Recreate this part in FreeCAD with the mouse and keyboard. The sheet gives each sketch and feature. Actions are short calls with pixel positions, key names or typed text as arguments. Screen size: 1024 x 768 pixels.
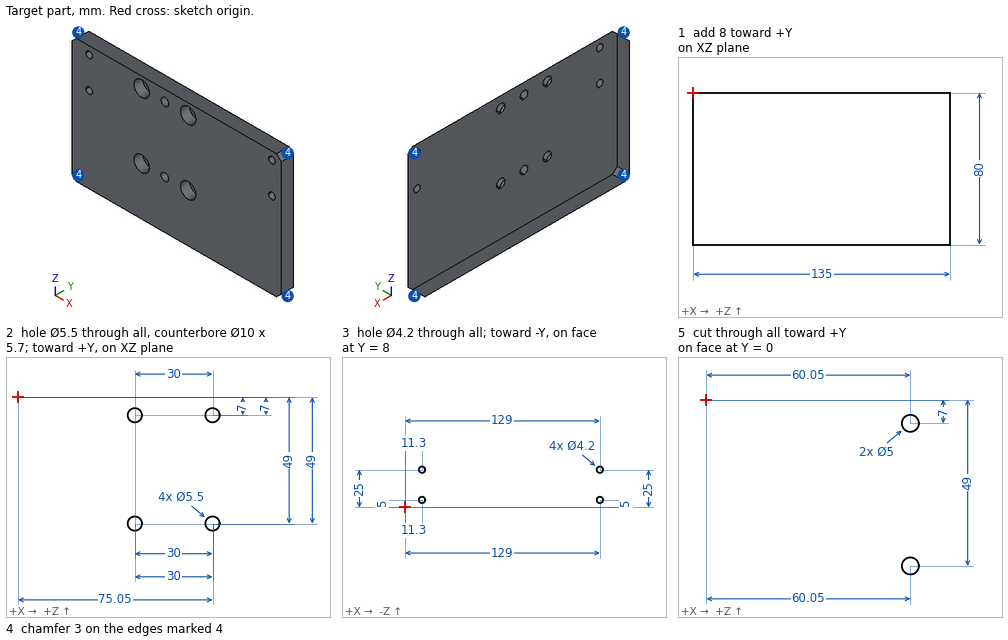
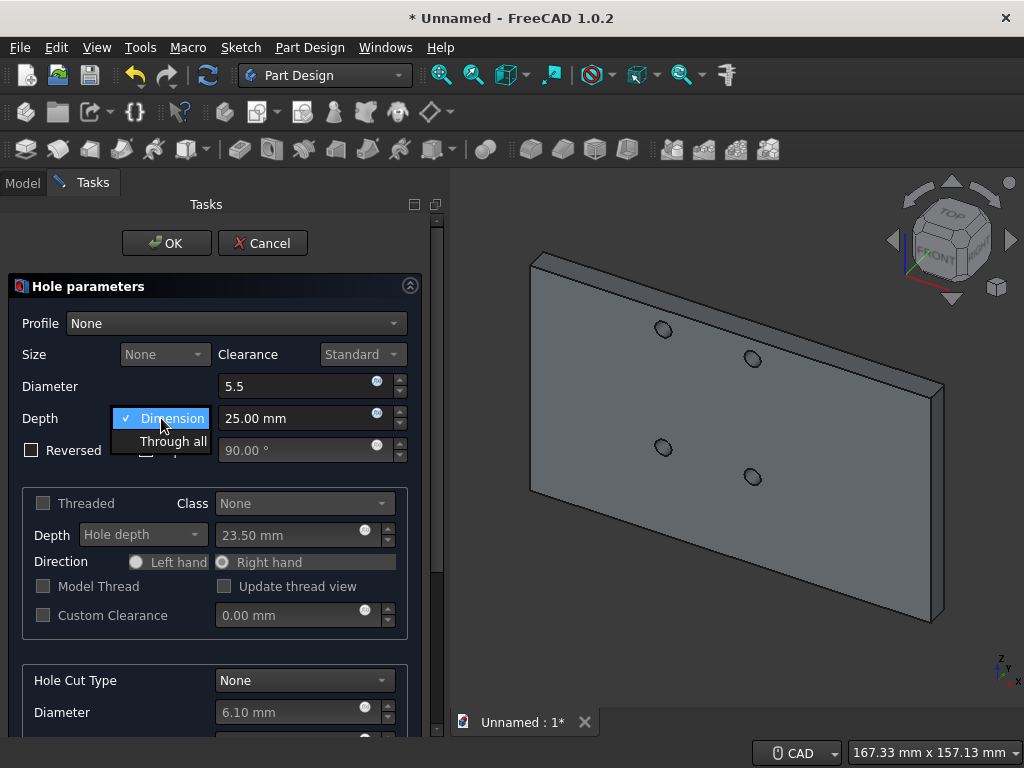
click(160, 442)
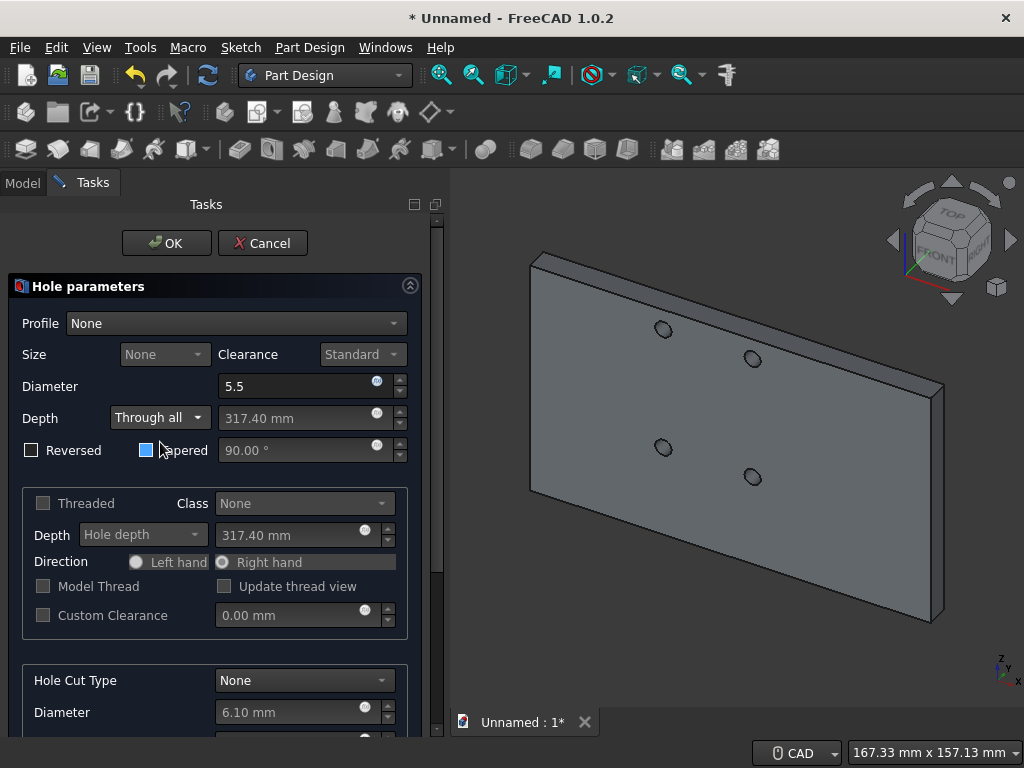
click(306, 680)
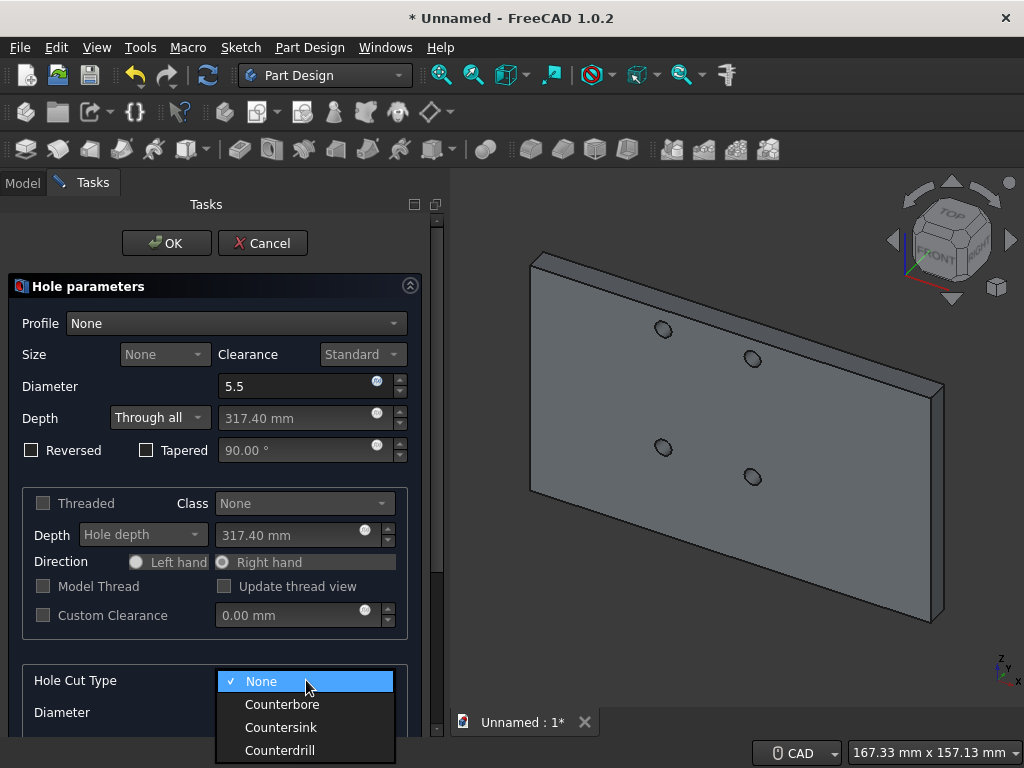
click(304, 704)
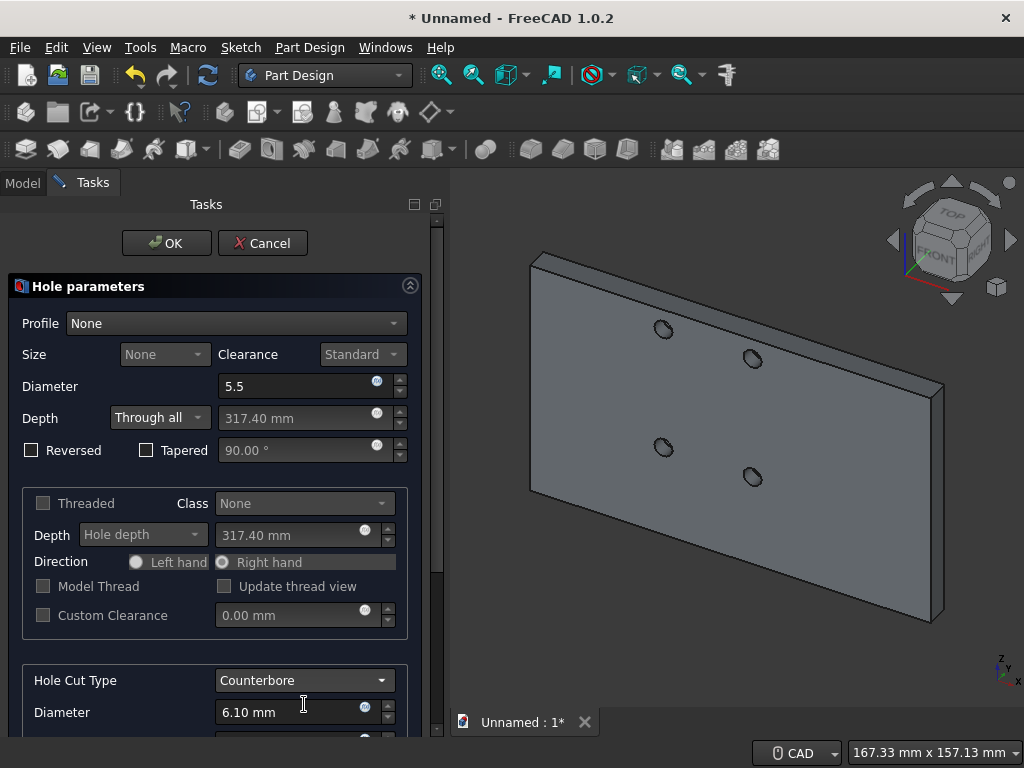
triple_click(298, 712)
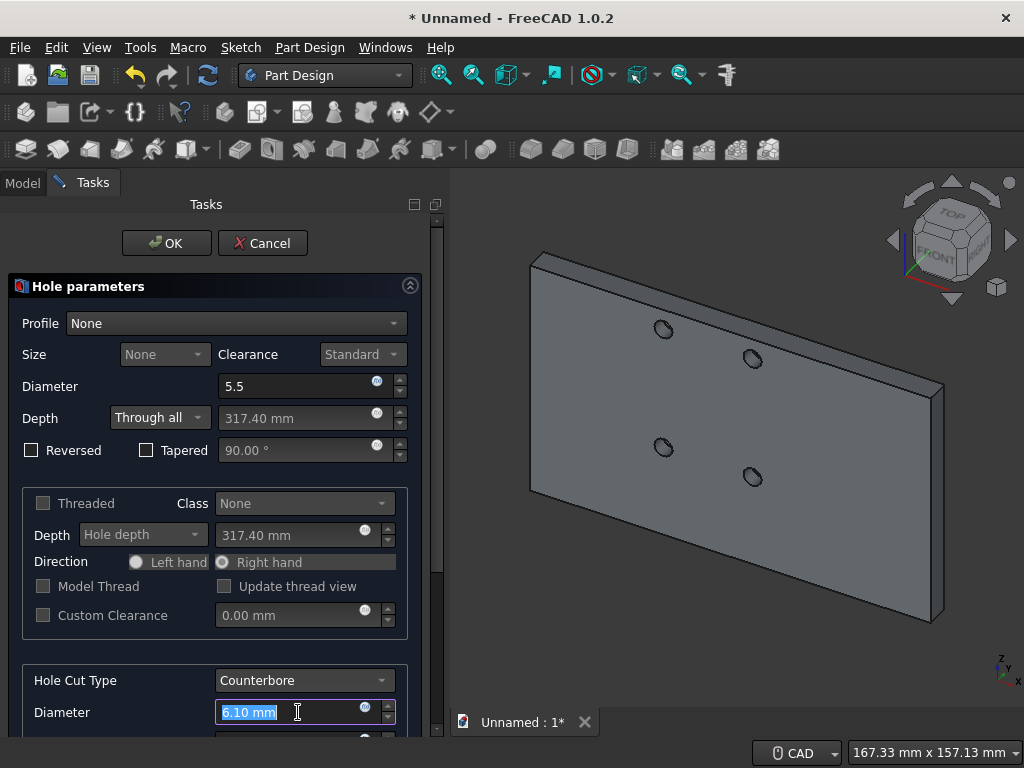
text(10)
key(Tab)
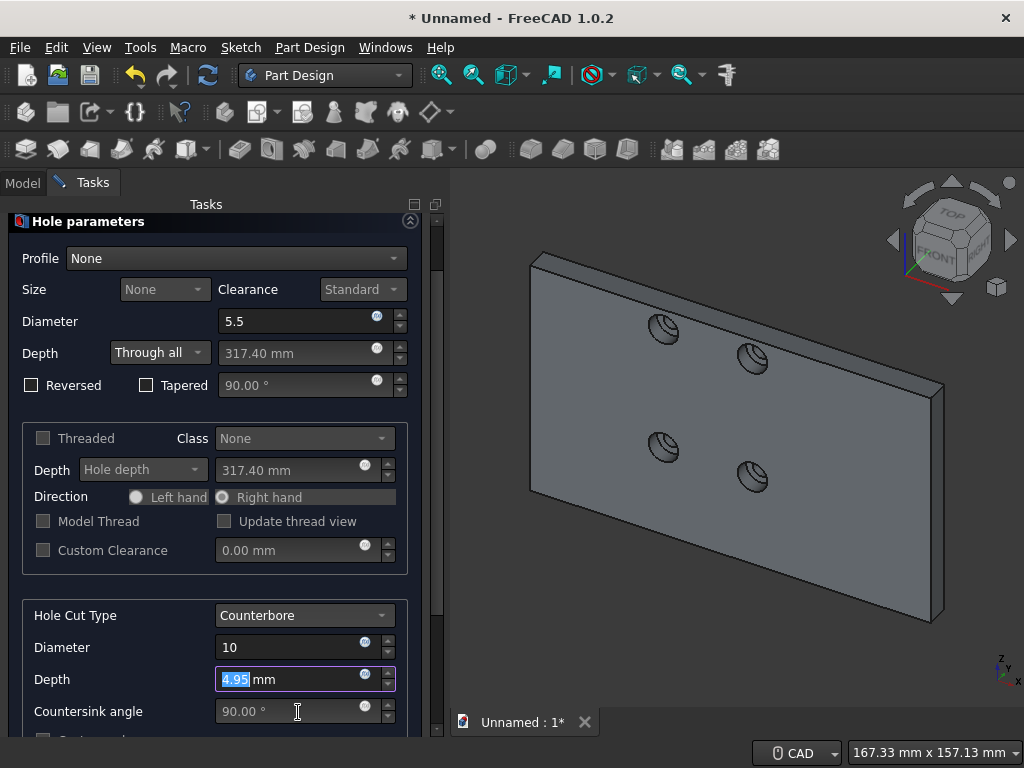
text(5.7)
key(Tab)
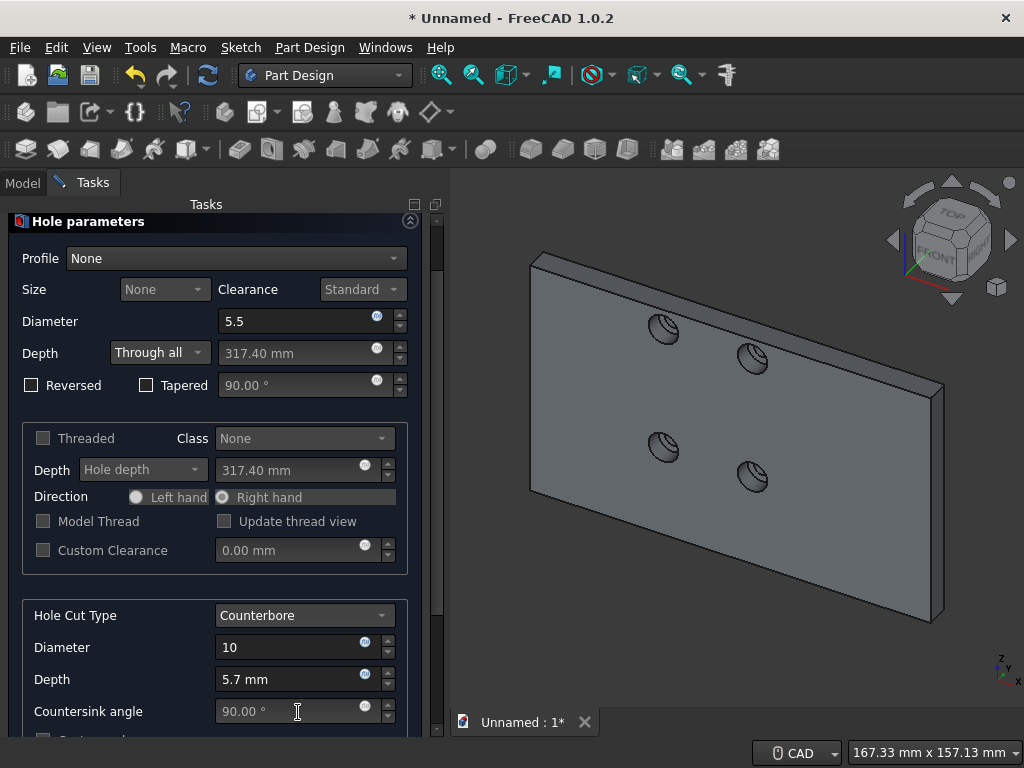
scroll(437, 475, up, 2)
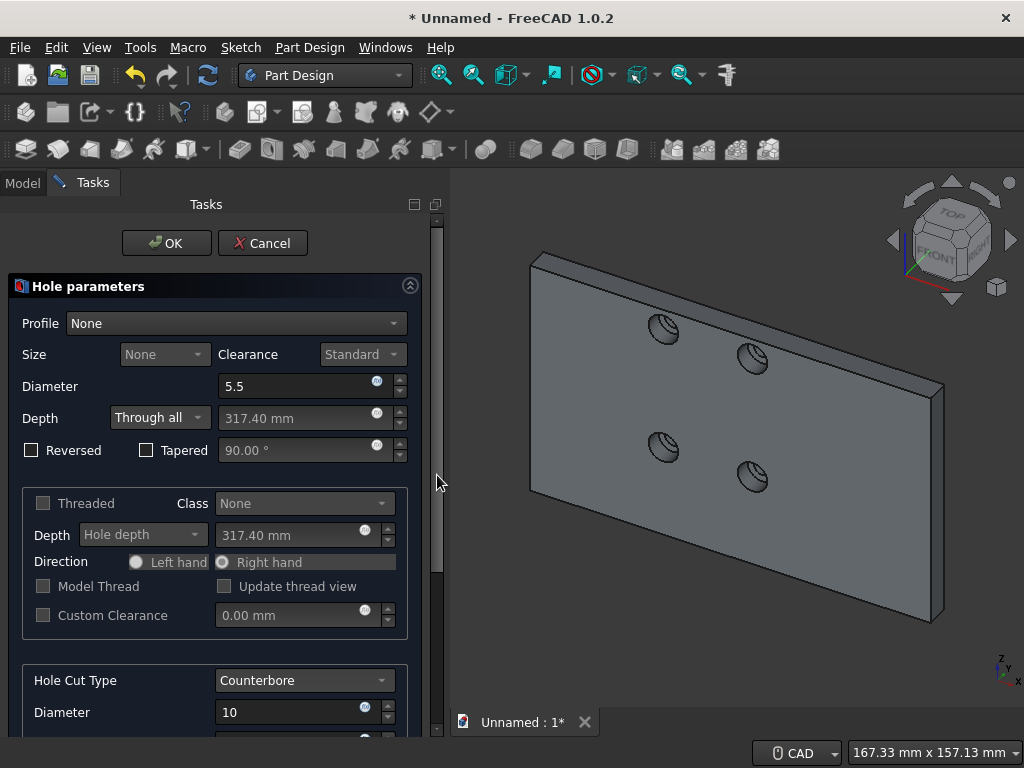
click(167, 243)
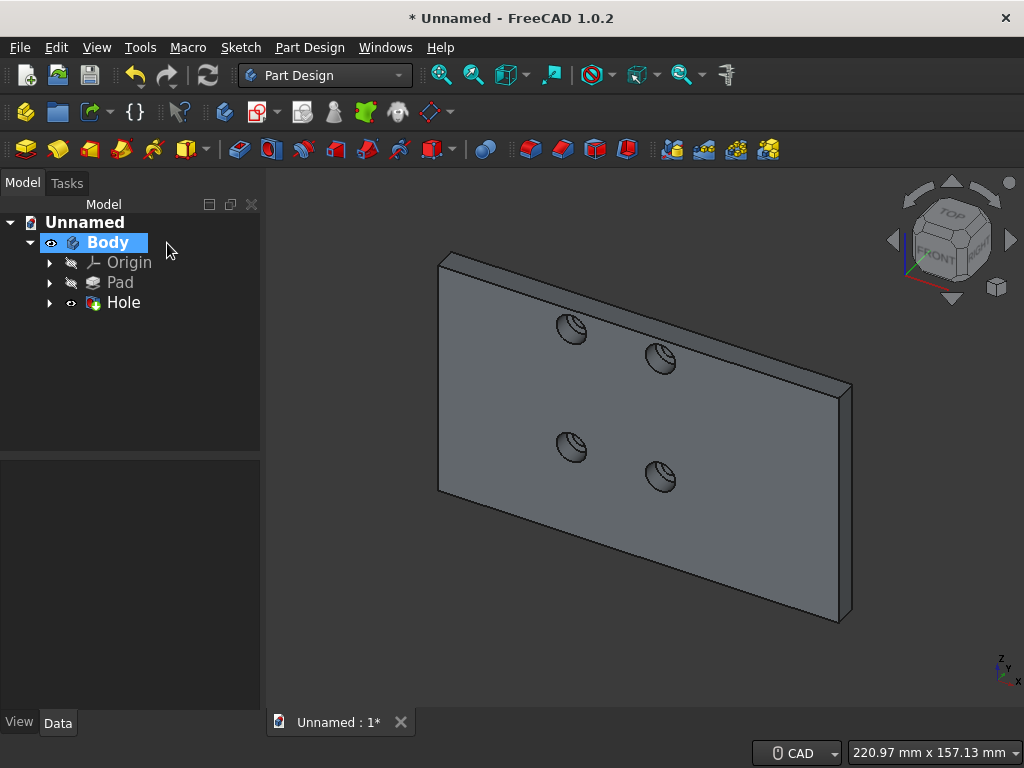
key(4)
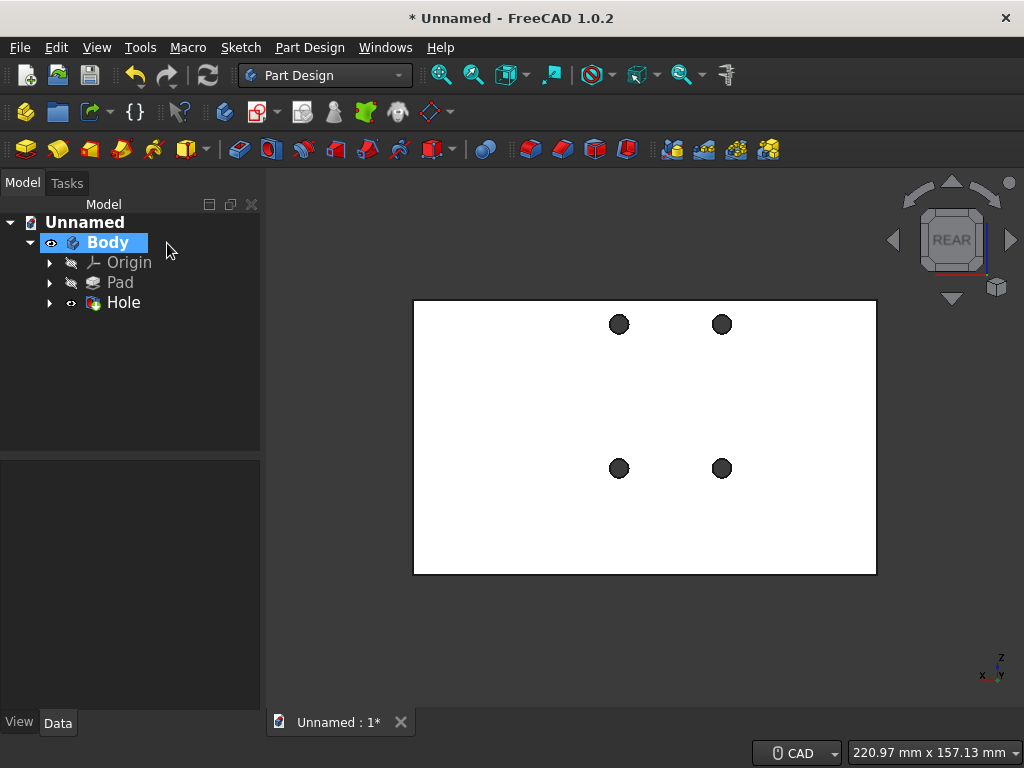
click(513, 436)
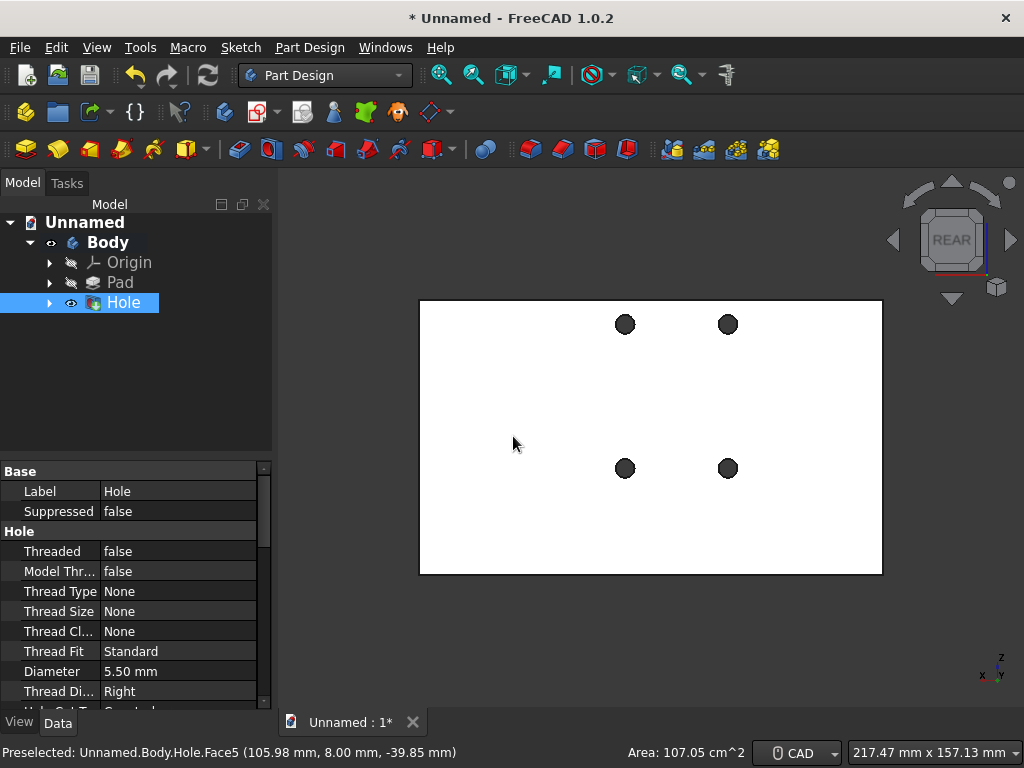
click(258, 112)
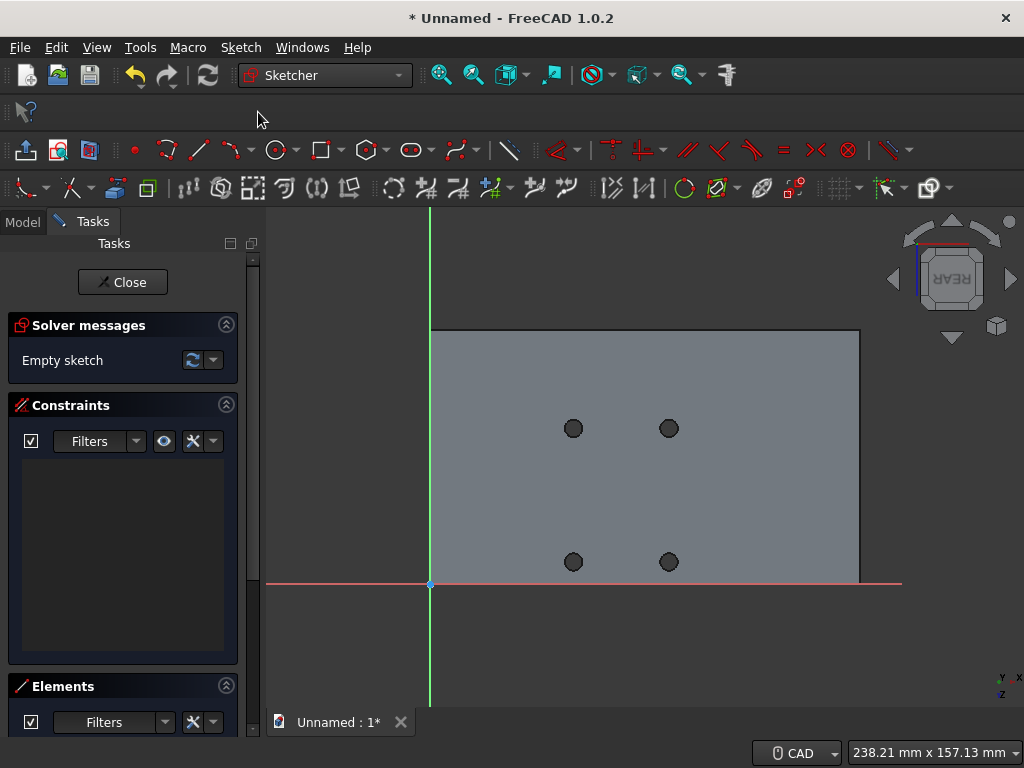
scroll(295, 235, down, 1)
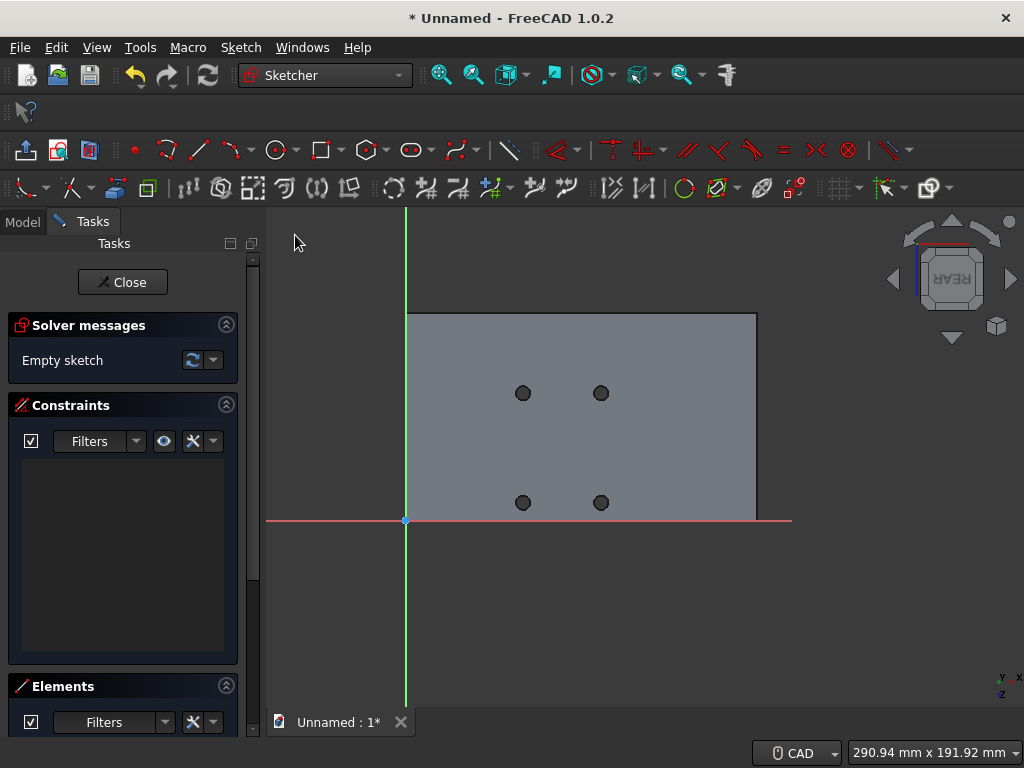
key(g)
key(c)